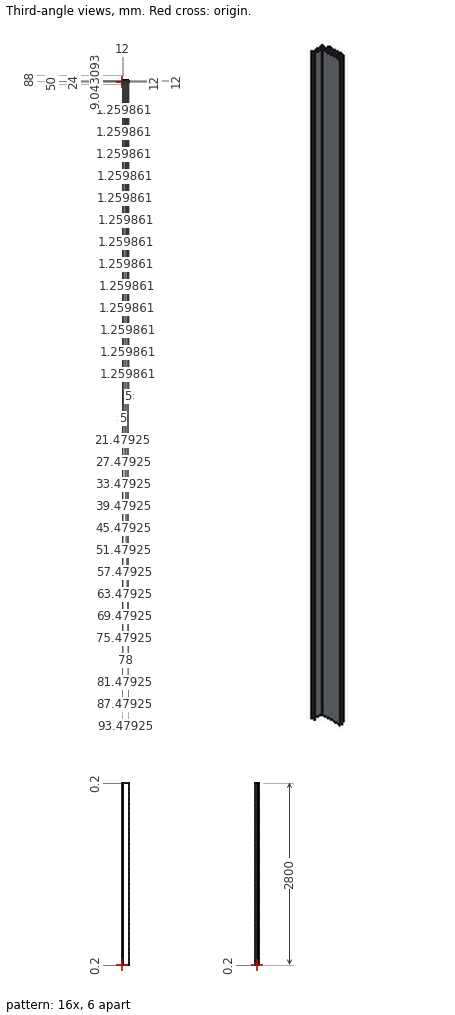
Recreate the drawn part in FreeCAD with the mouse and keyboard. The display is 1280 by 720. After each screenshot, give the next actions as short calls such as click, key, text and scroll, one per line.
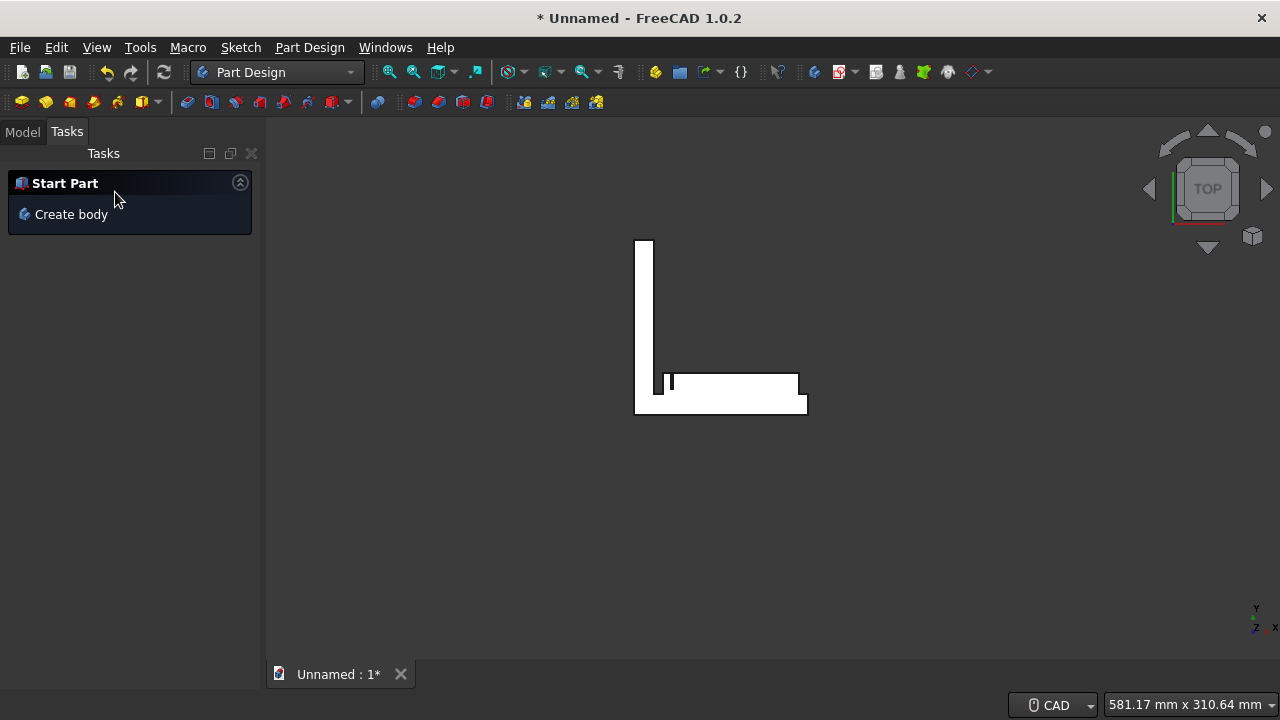
click(390, 72)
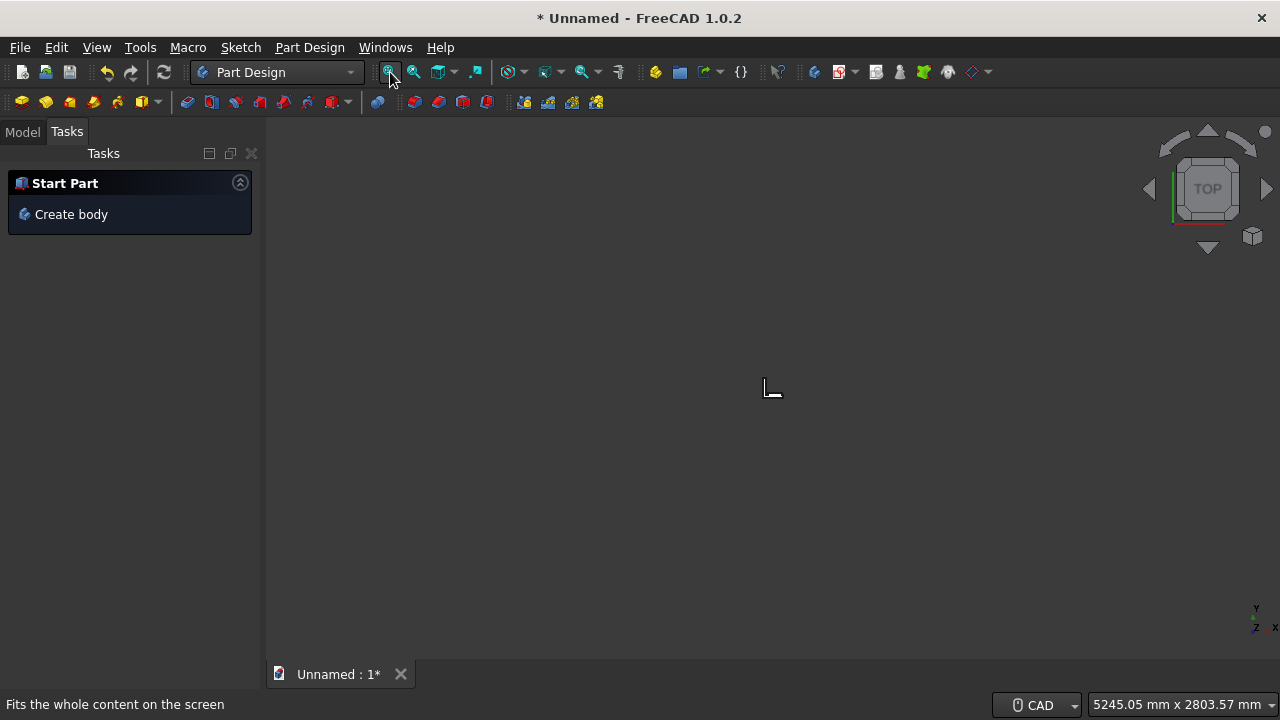
click(23, 131)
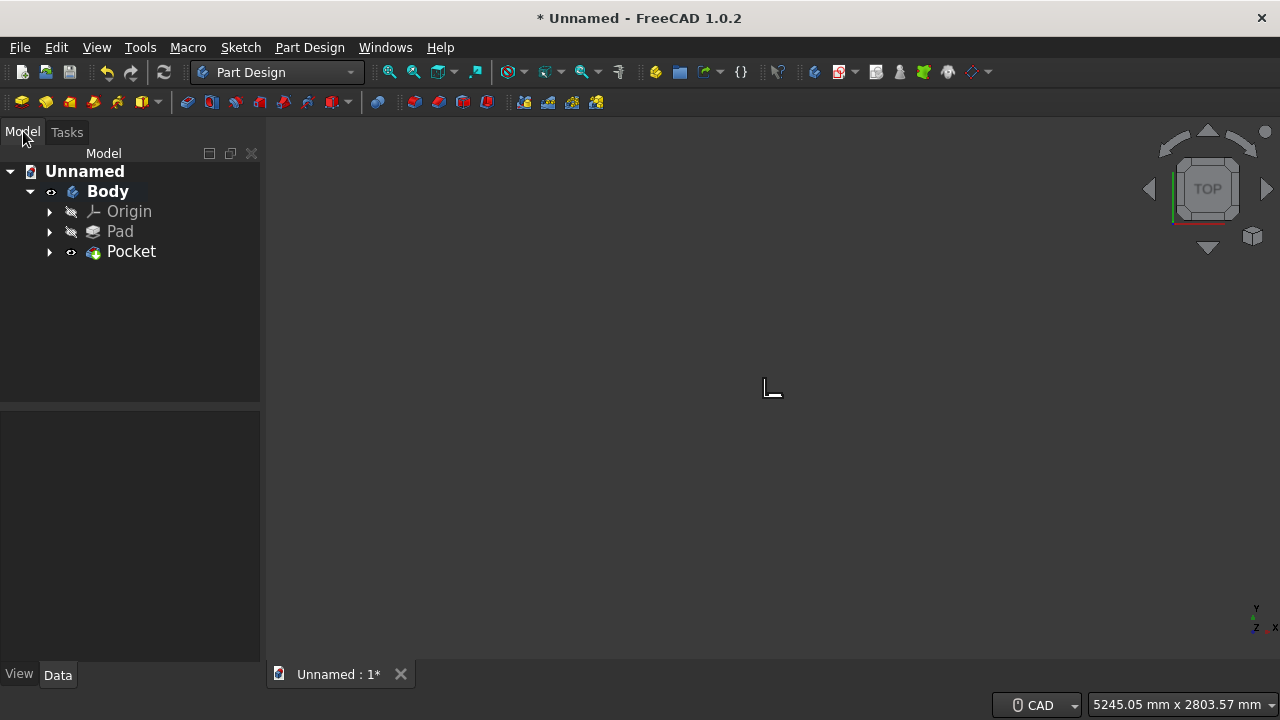
click(116, 252)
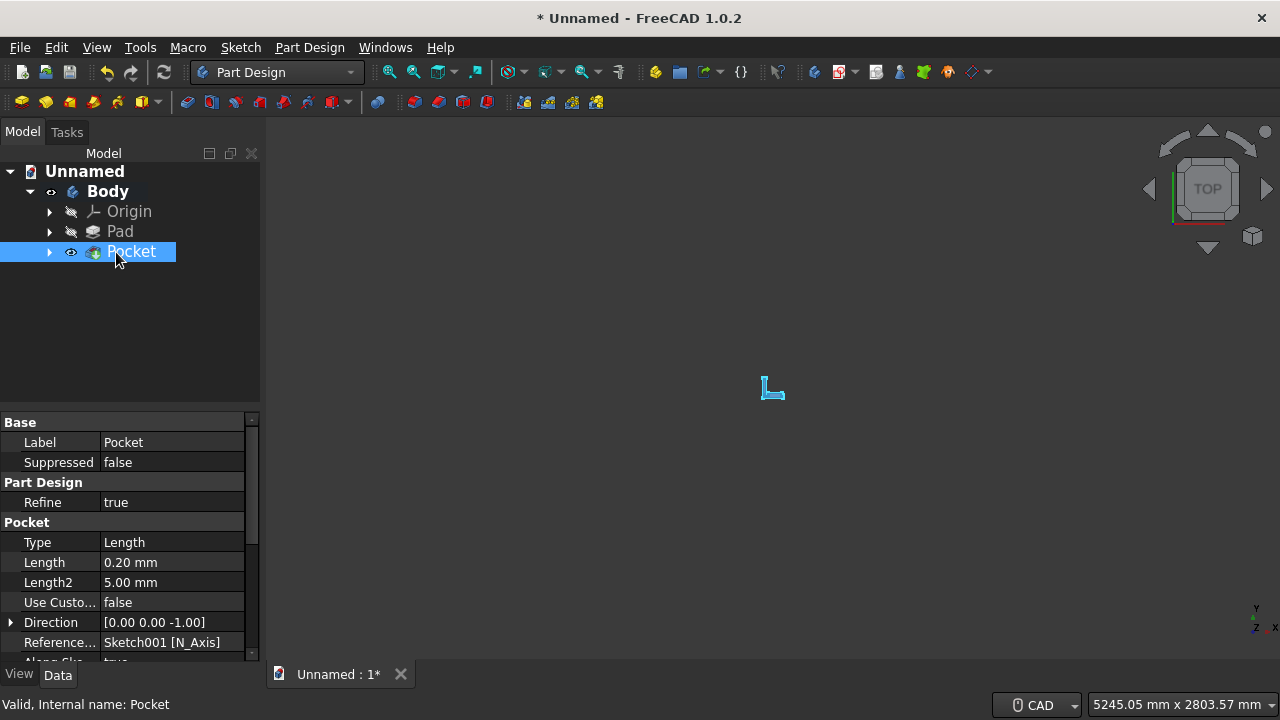
click(548, 102)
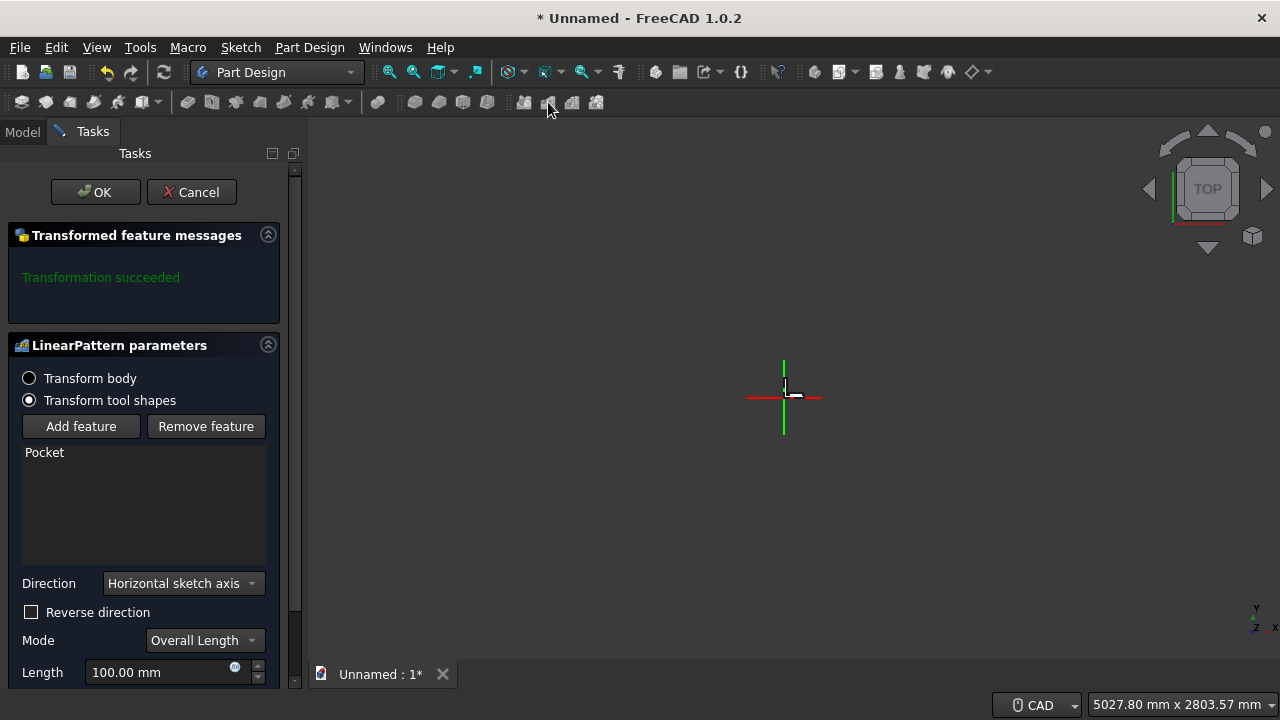
click(184, 584)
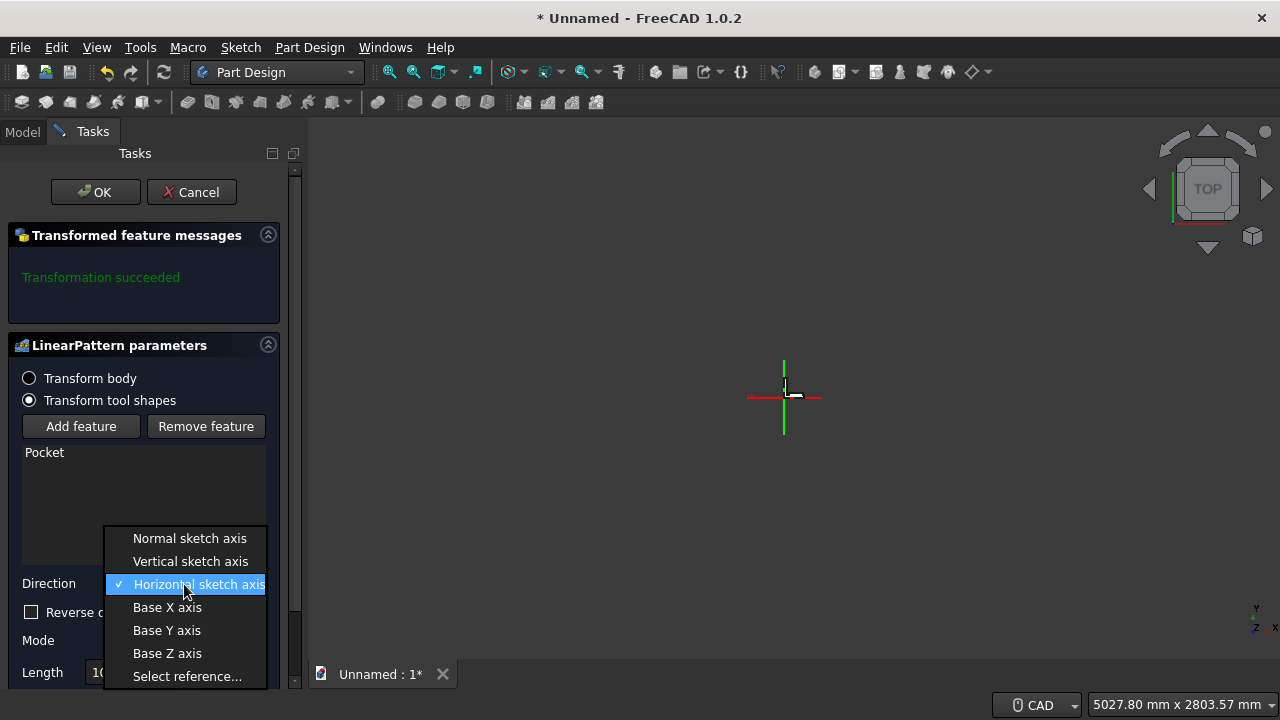
click(184, 608)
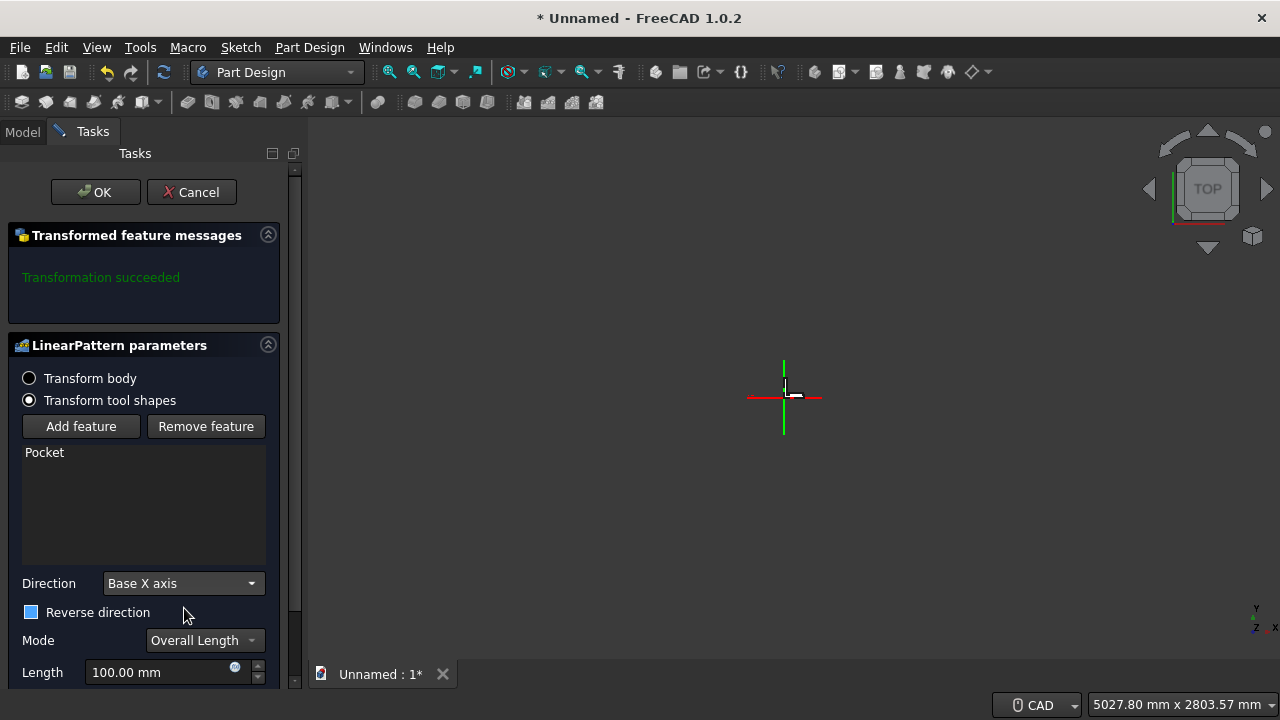
click(206, 640)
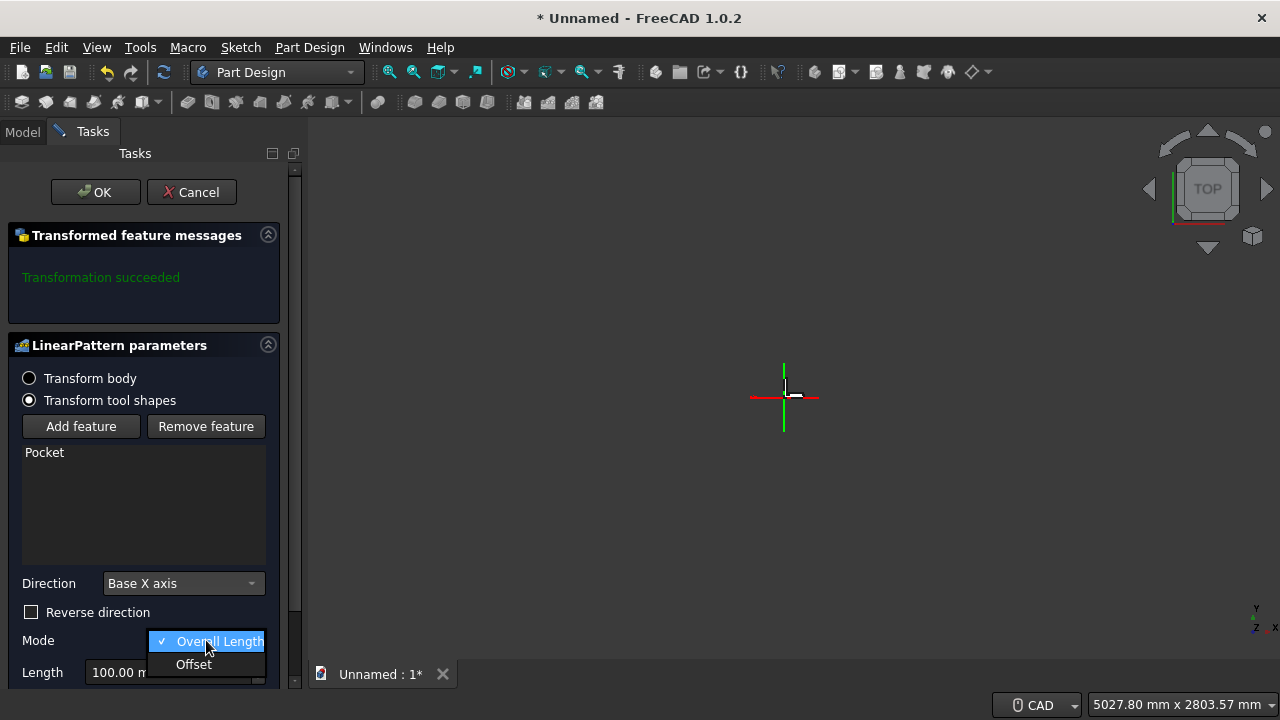
click(206, 664)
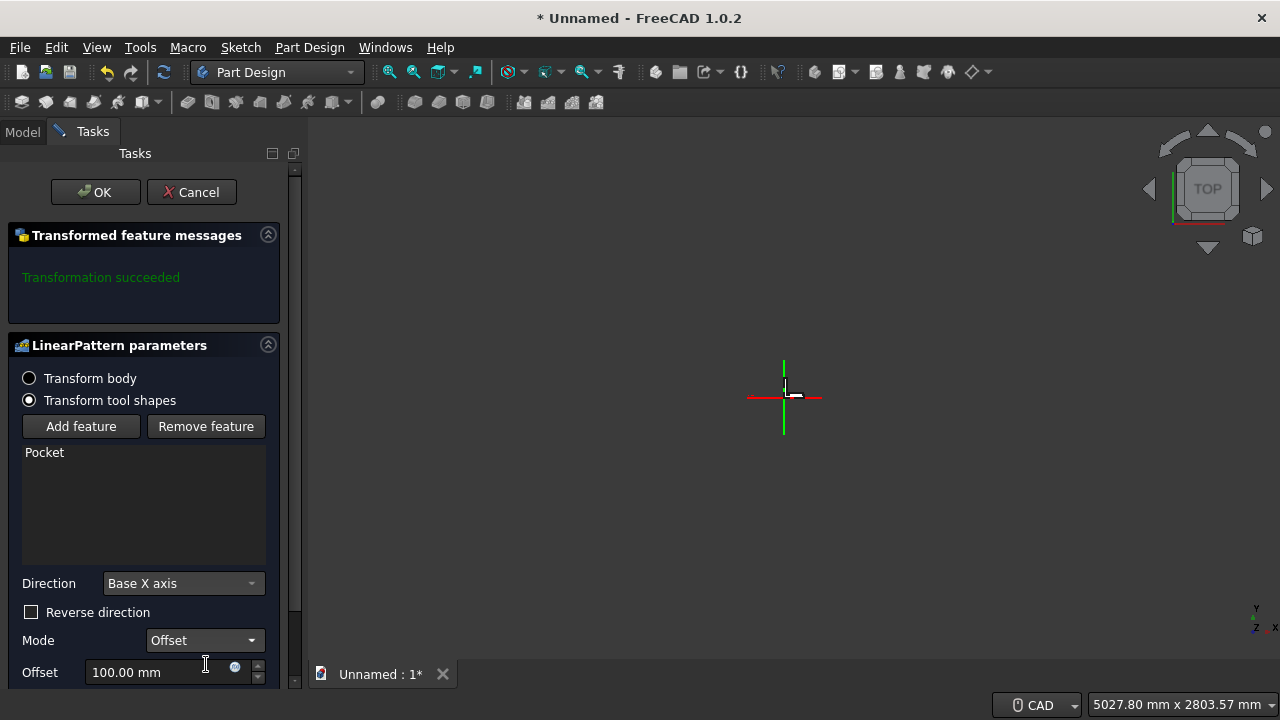
triple_click(168, 672)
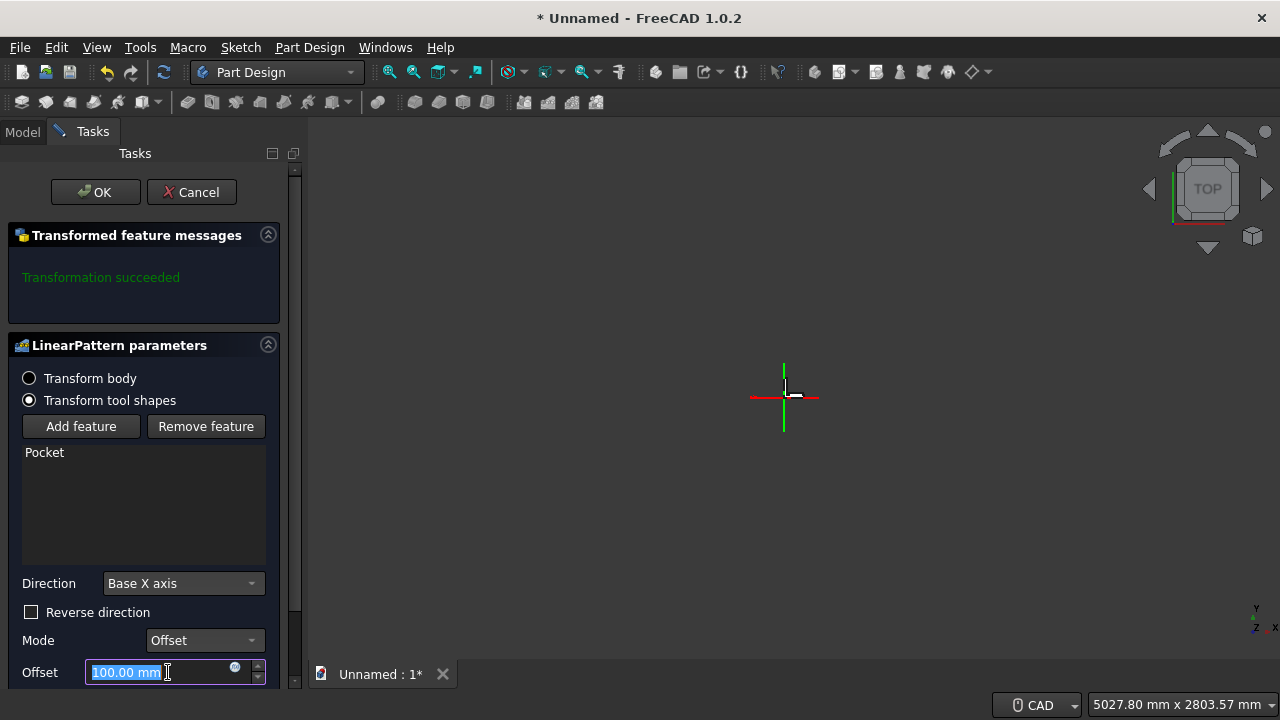
text(6)
key(Tab)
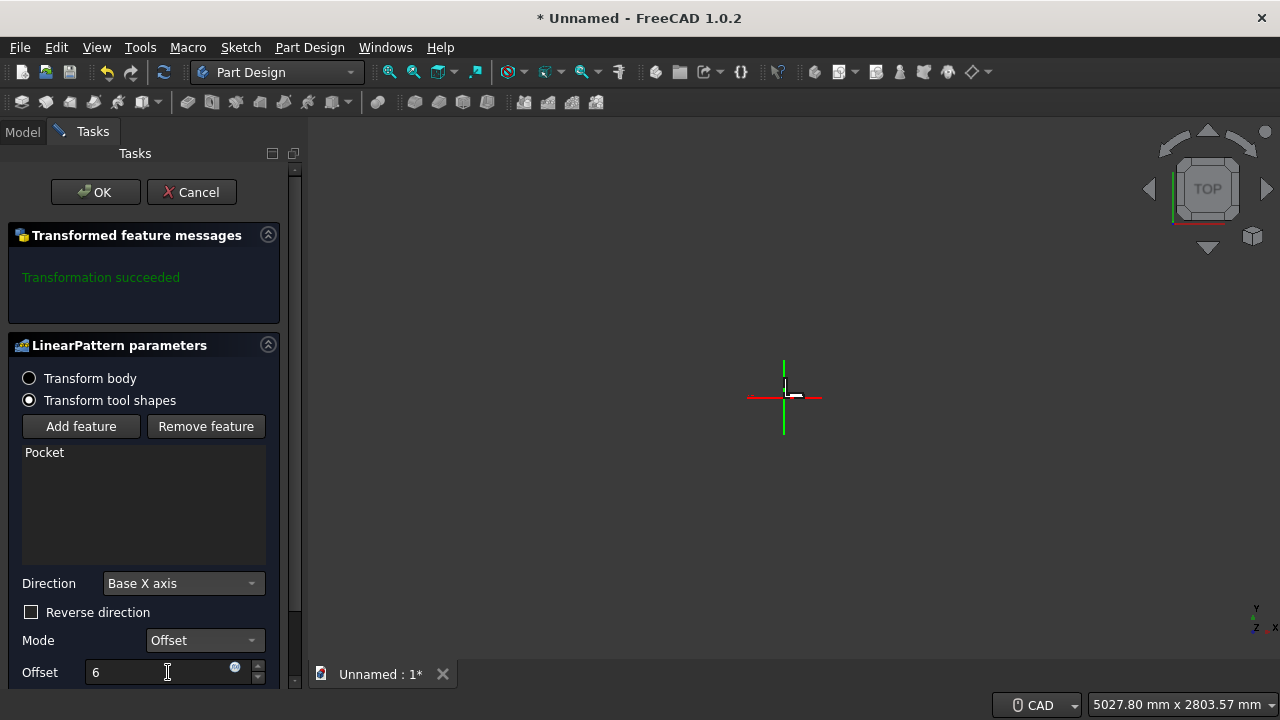
scroll(295, 426, down, 2)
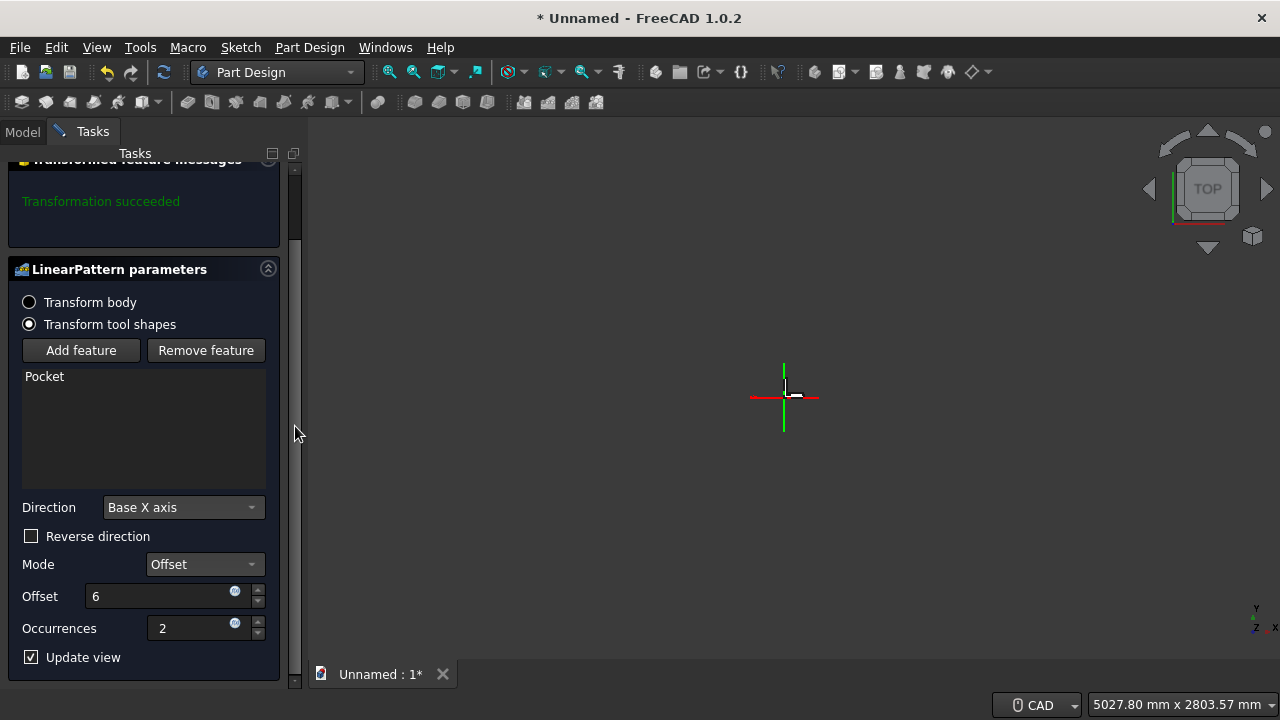
triple_click(198, 628)